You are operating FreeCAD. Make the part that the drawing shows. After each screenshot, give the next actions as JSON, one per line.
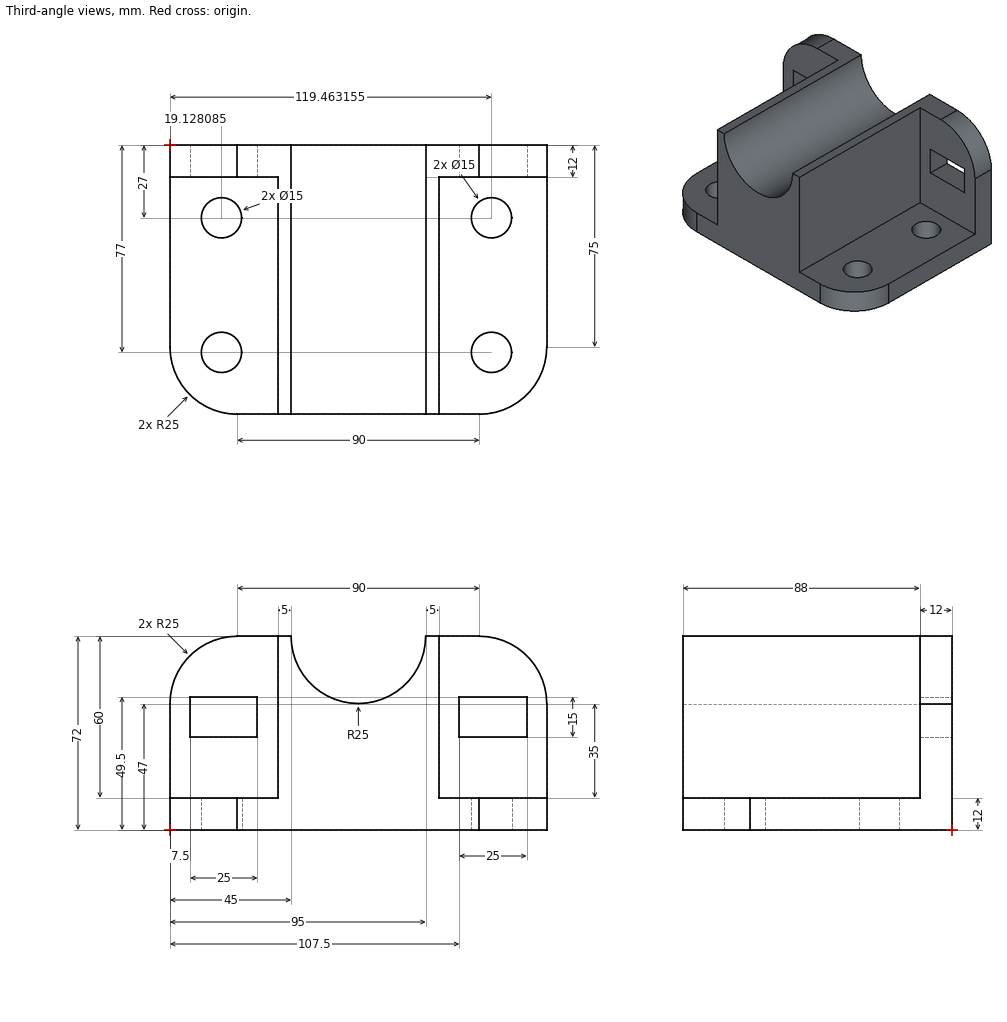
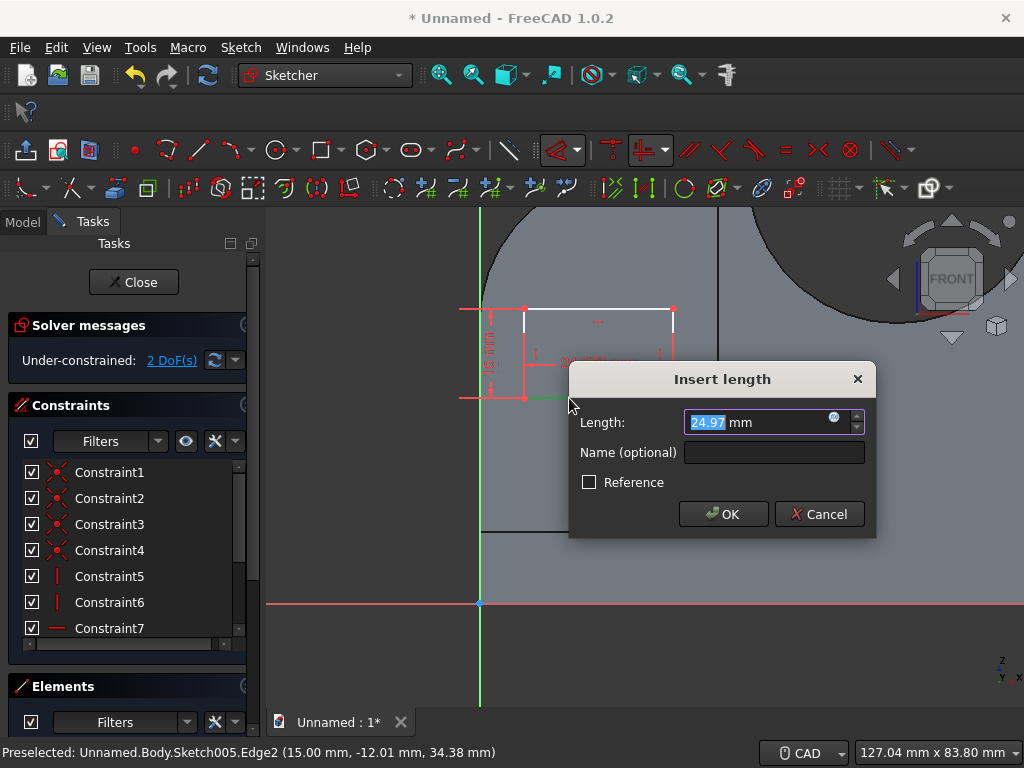
{"action": "type", "text": "25"}
{"action": "key", "text": "Return"}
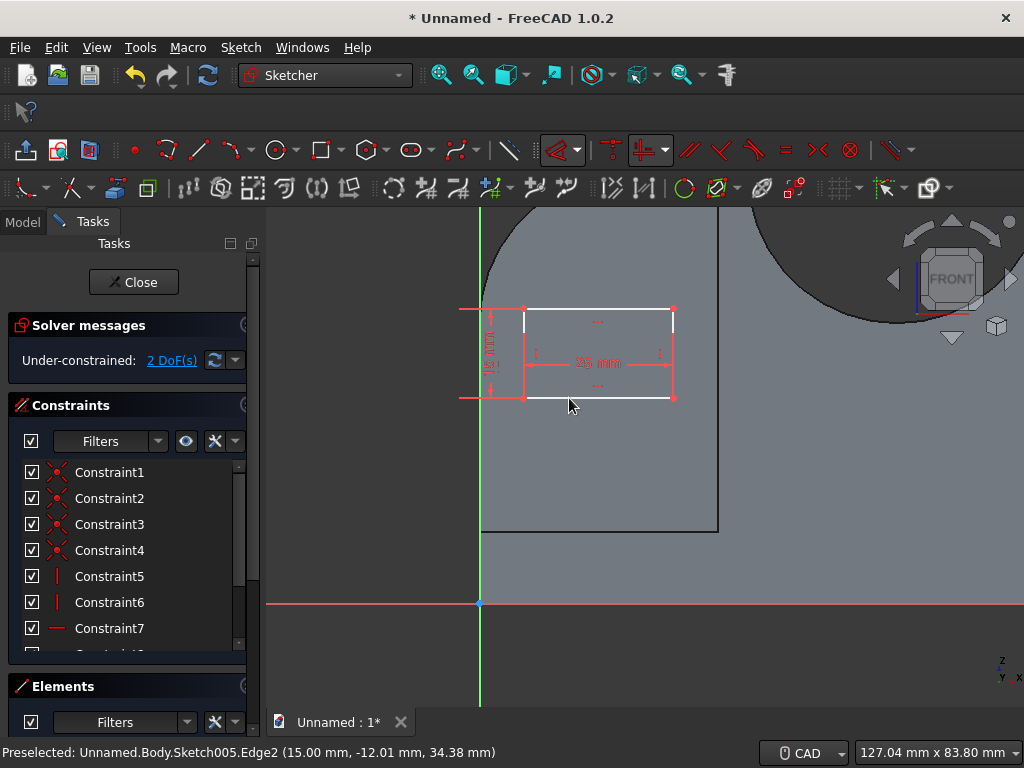
{"action": "left_click", "coordinate": [524, 309]}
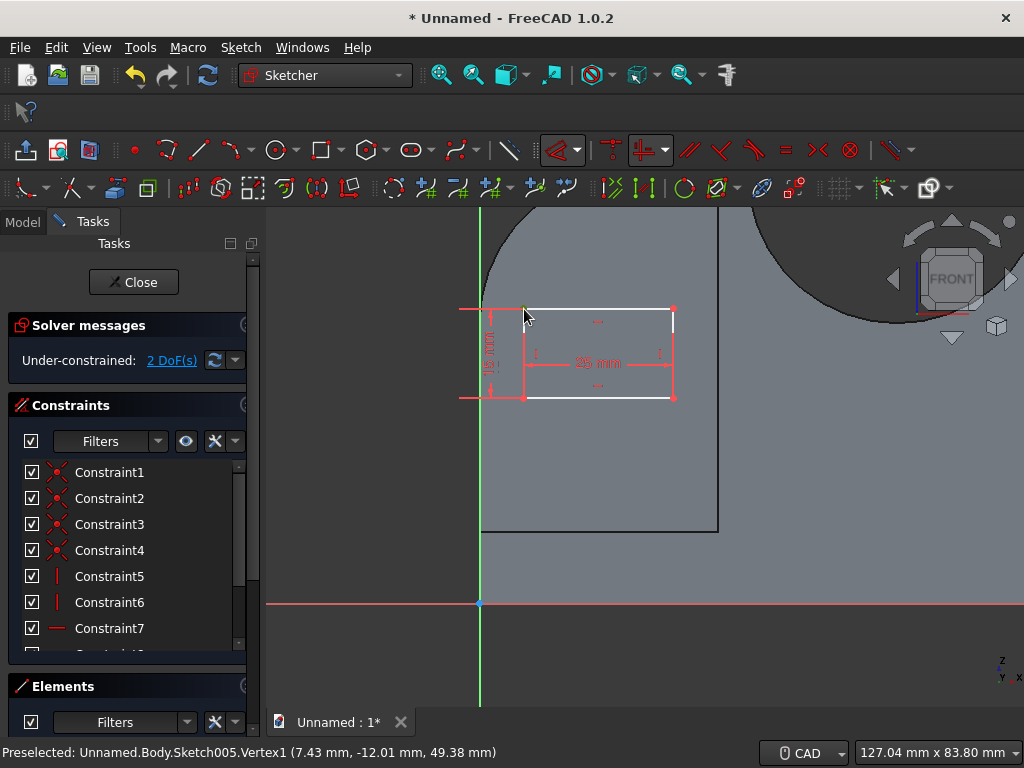
{"action": "left_click", "coordinate": [580, 150]}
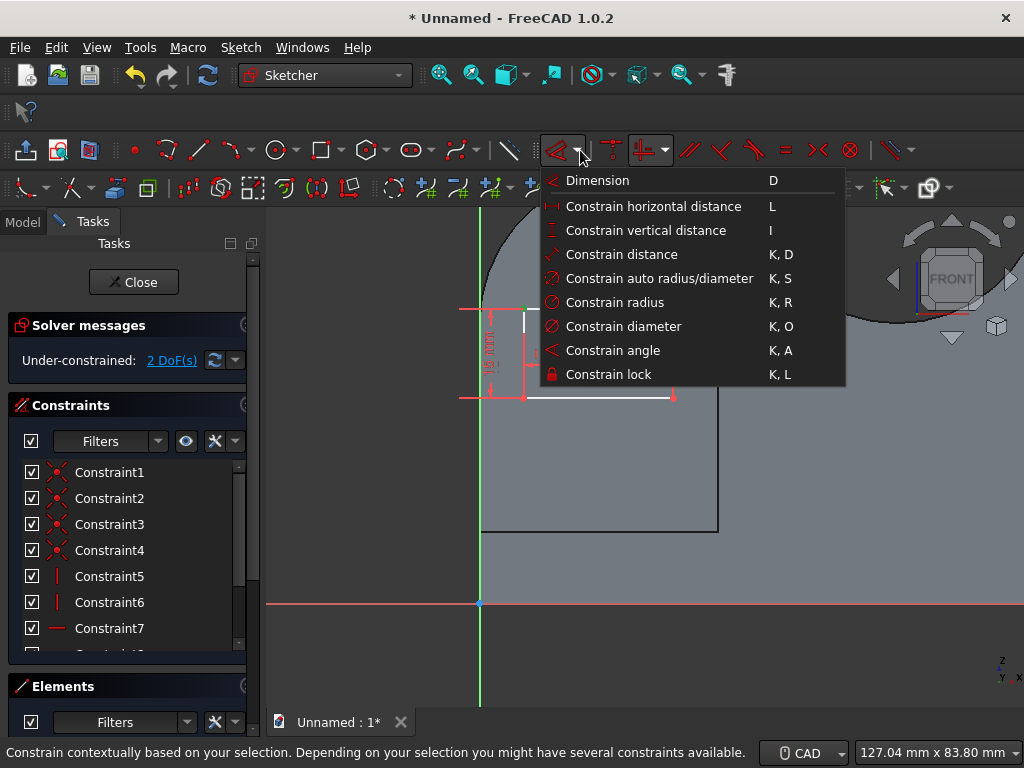
{"action": "left_click", "coordinate": [693, 206]}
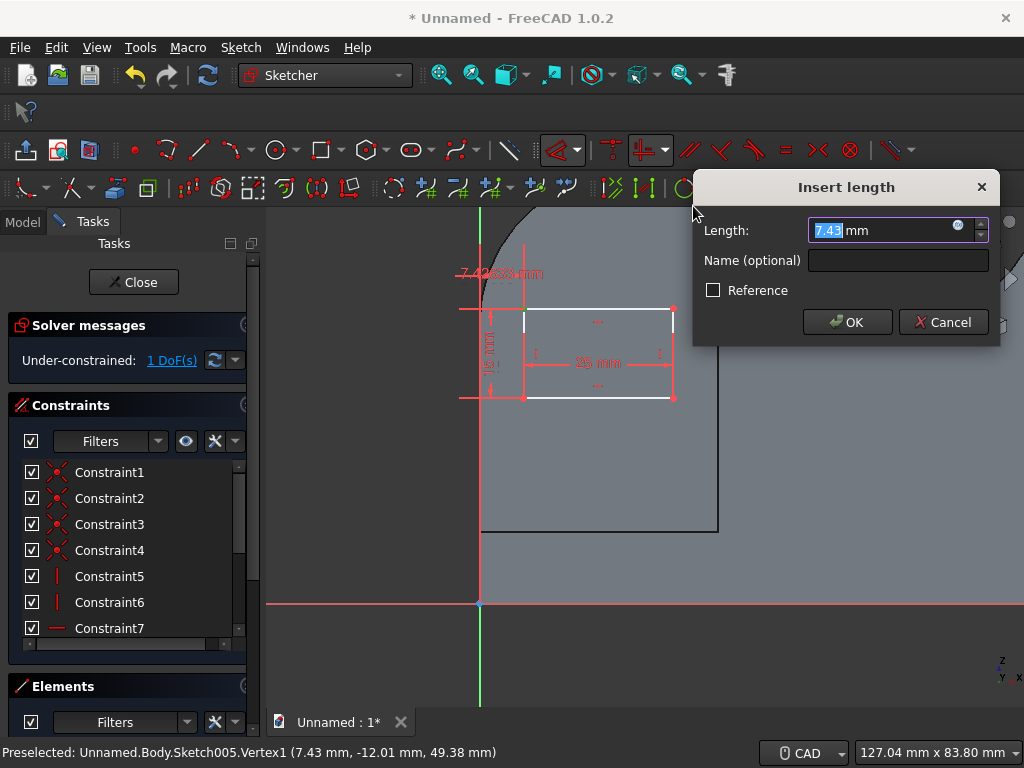
{"action": "type", "text": "7.5"}
{"action": "key", "text": "Return"}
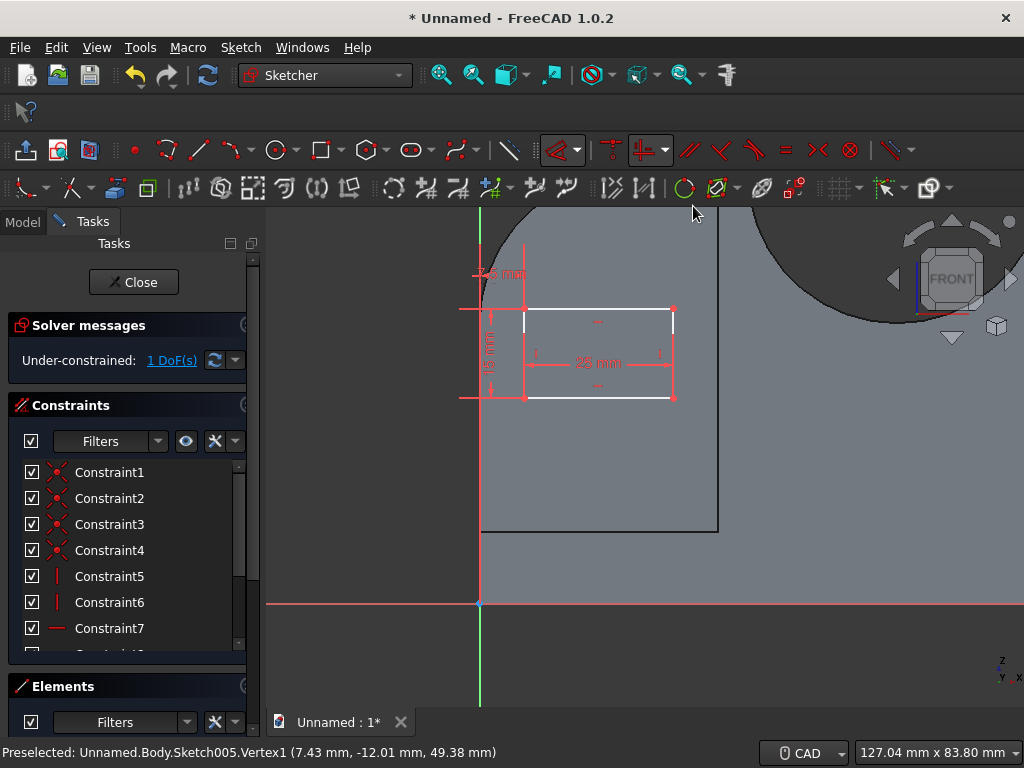
{"action": "left_click", "coordinate": [524, 309]}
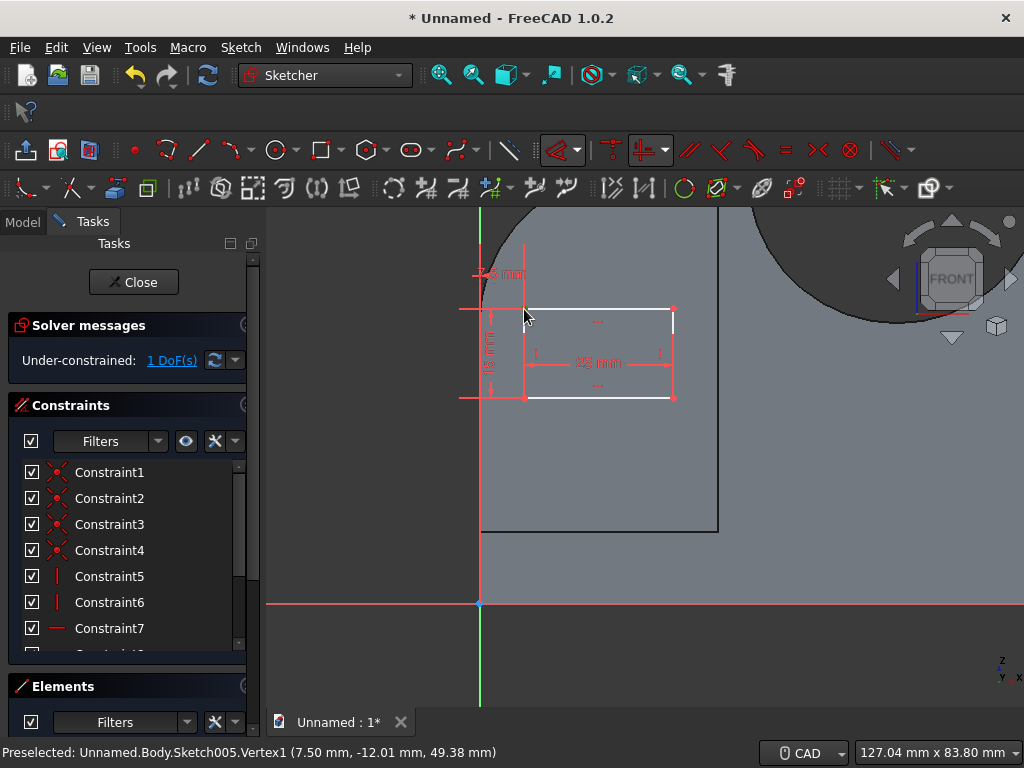
{"action": "key", "text": "i"}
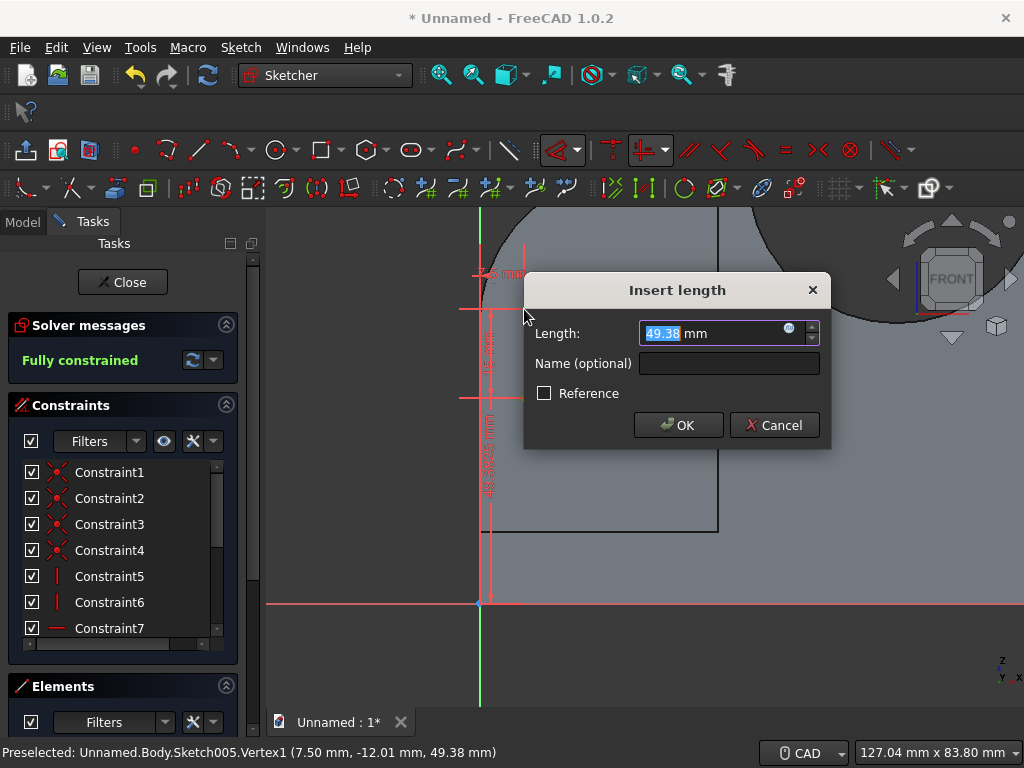
{"action": "type", "text": "49.5"}
{"action": "key", "text": "Return"}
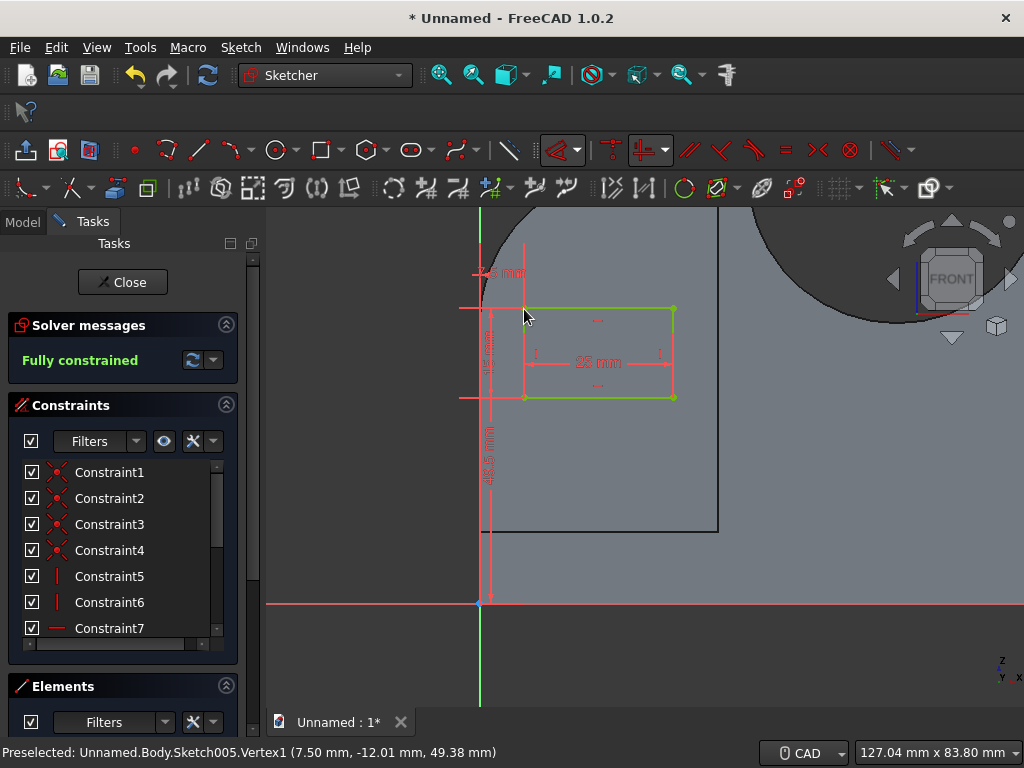
{"action": "left_click", "coordinate": [123, 282]}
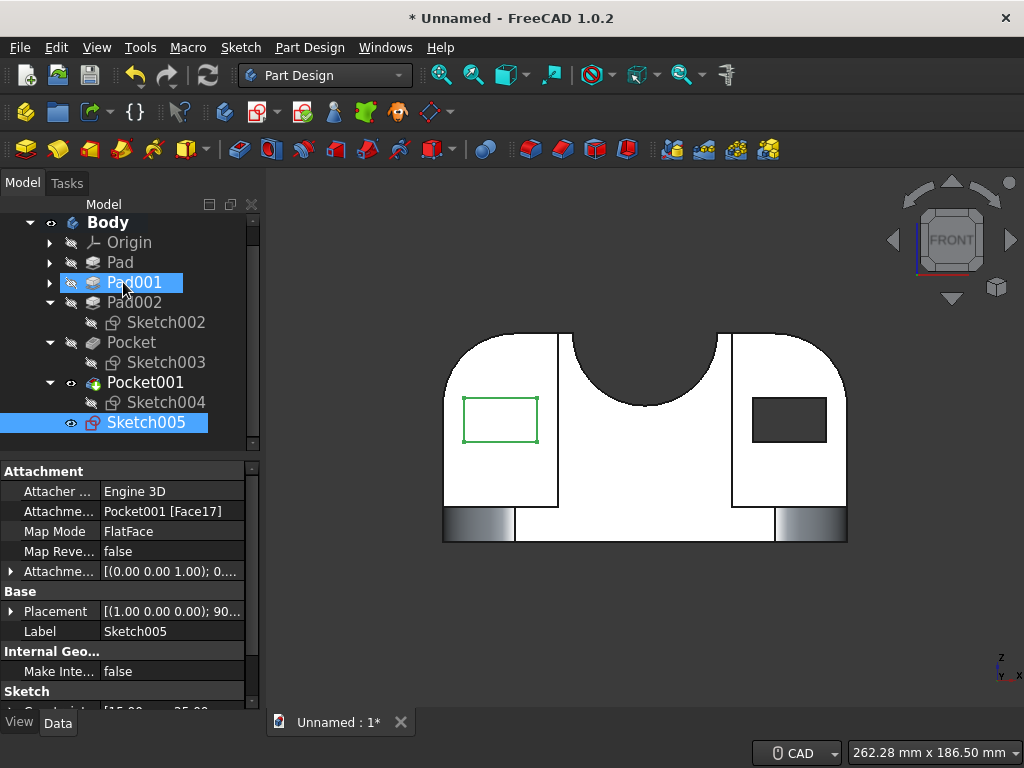
{"action": "left_click", "coordinate": [240, 150]}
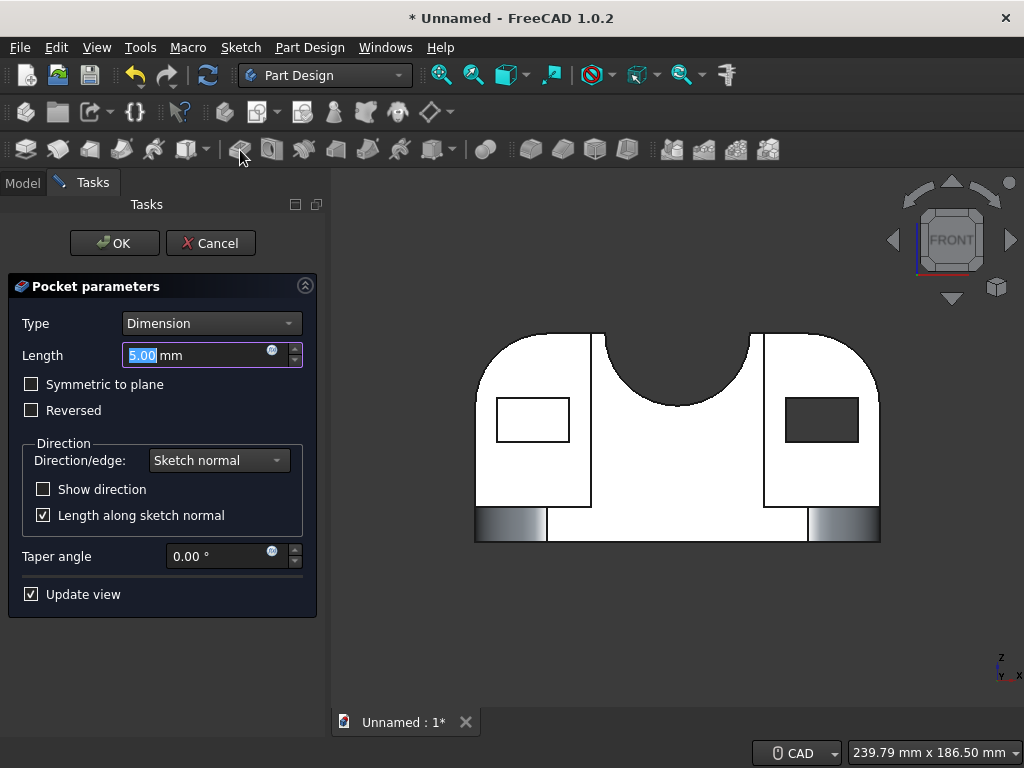
{"action": "type", "text": "12"}
{"action": "key", "text": "Tab"}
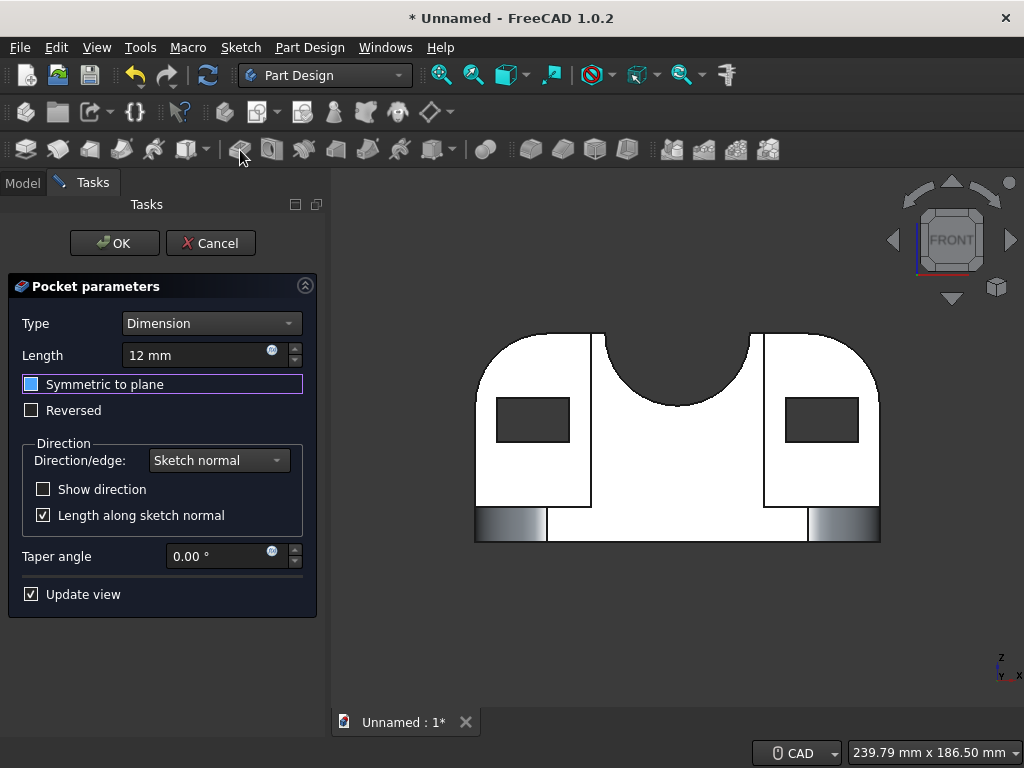
{"action": "left_click", "coordinate": [115, 243]}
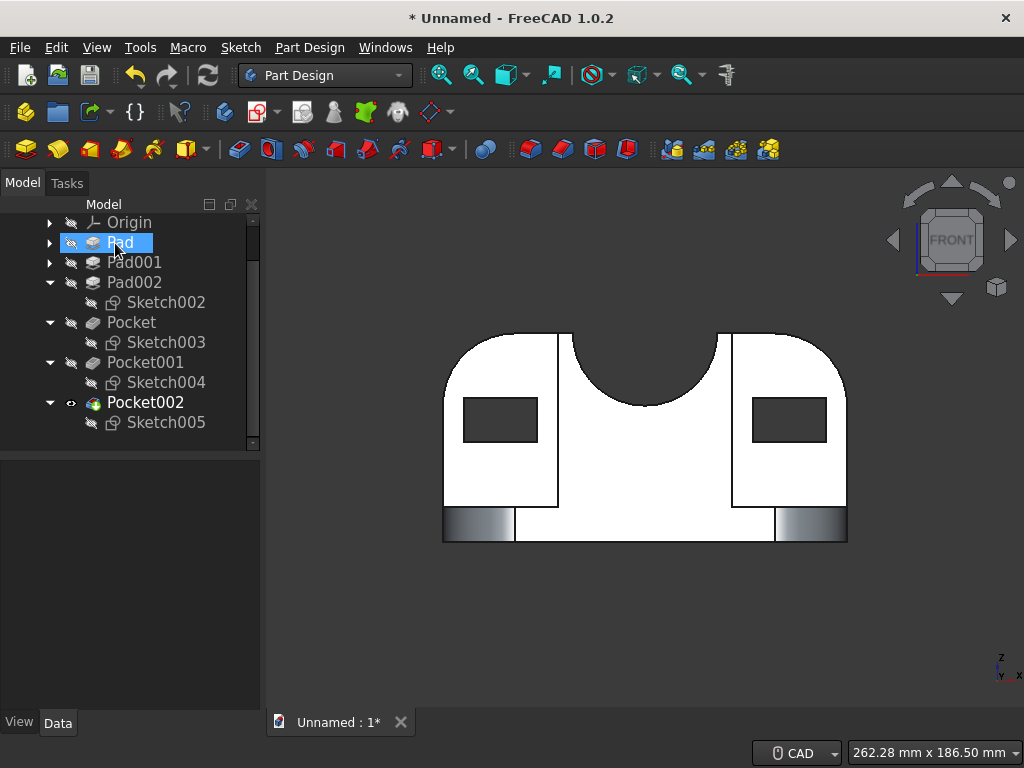
{"action": "key", "text": "0"}